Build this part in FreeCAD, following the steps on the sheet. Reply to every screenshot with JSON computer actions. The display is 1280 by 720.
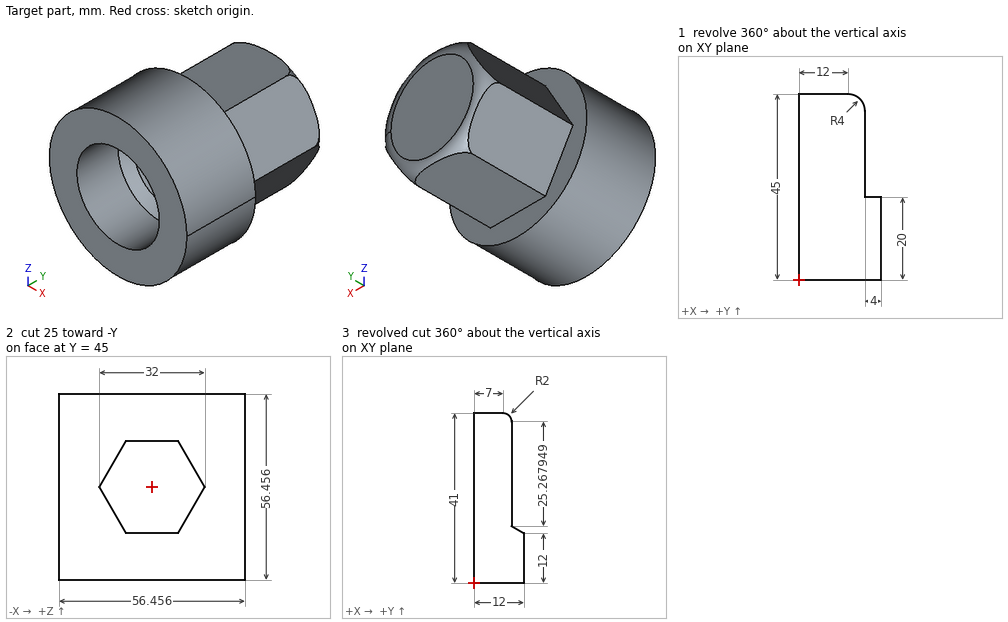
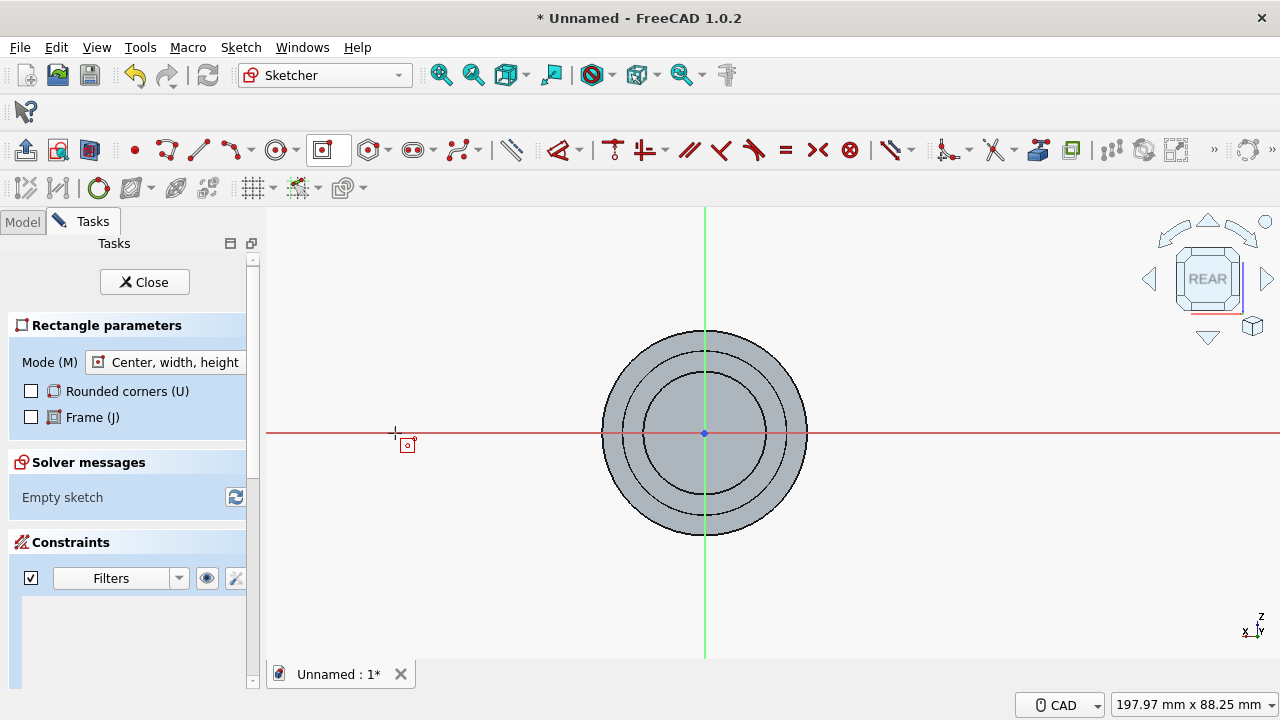
{"action": "left_click", "coordinate": [705, 433]}
{"action": "mouse_move", "coordinate": [849, 289]}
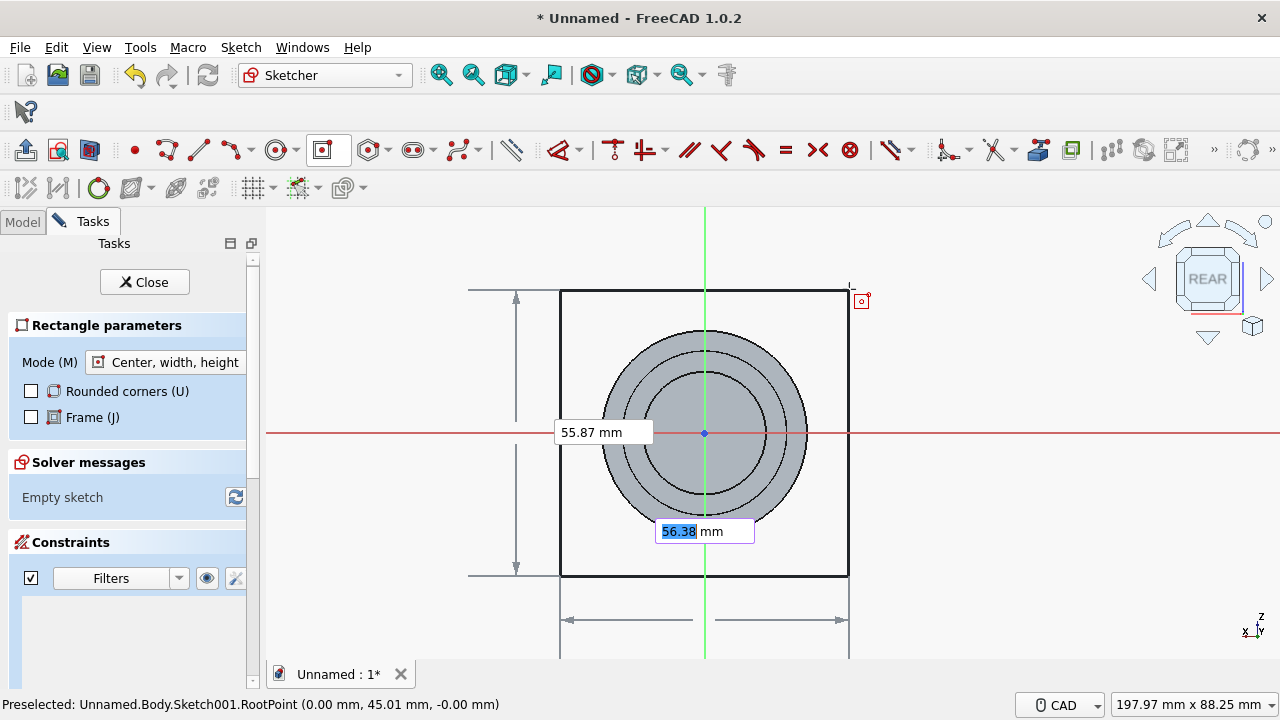
{"action": "type", "text": "56.456"}
{"action": "key", "text": "Tab"}
{"action": "type", "text": "56.456"}
{"action": "key", "text": "Return"}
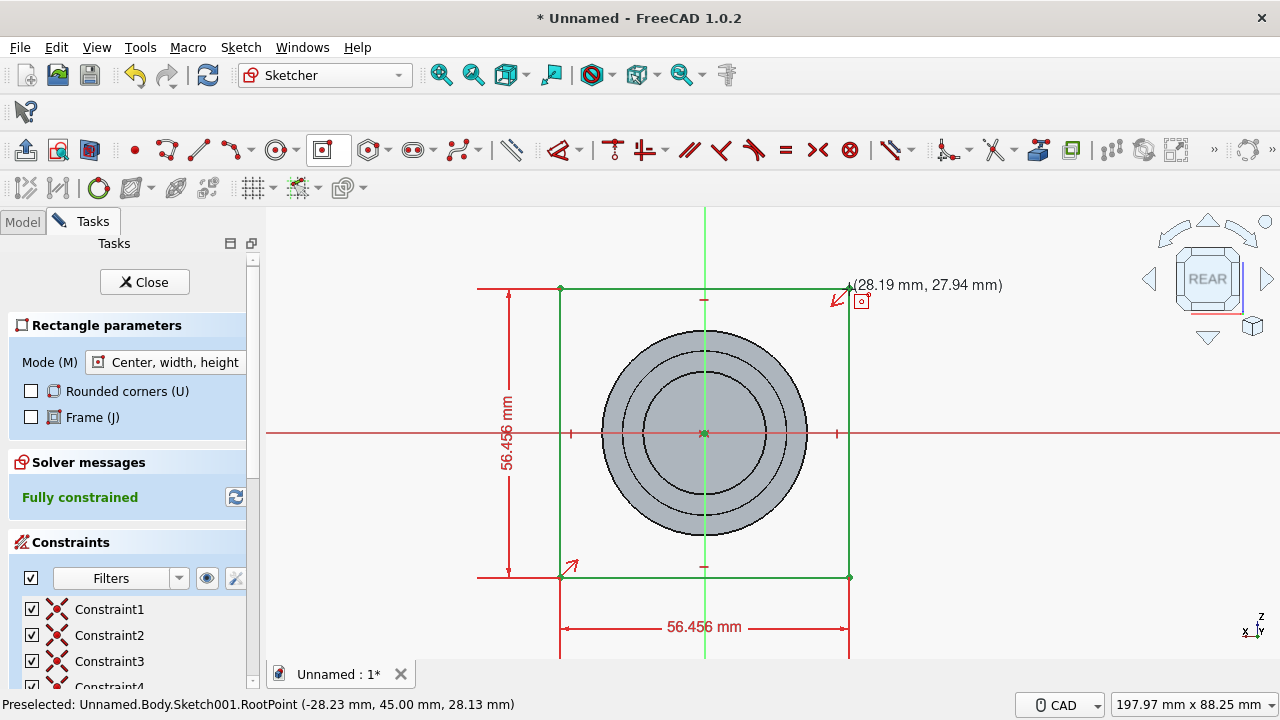
{"action": "key", "text": "g p 6"}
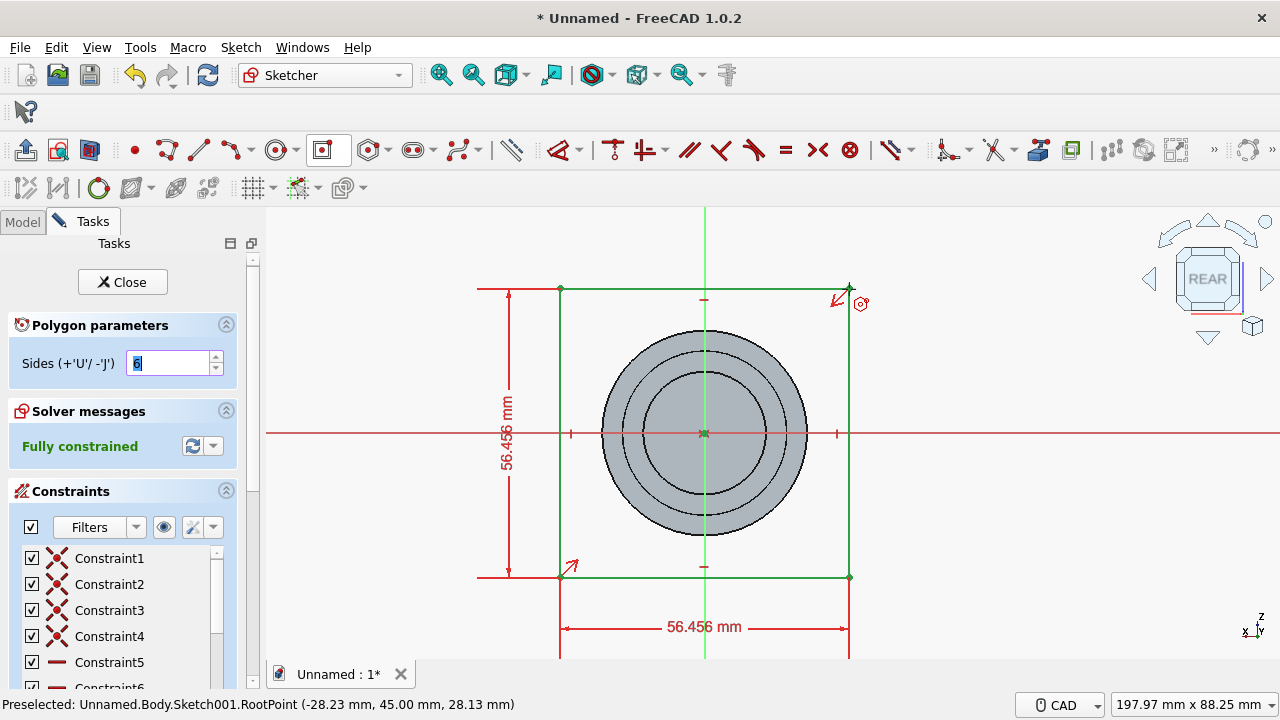
{"action": "left_click", "coordinate": [705, 433]}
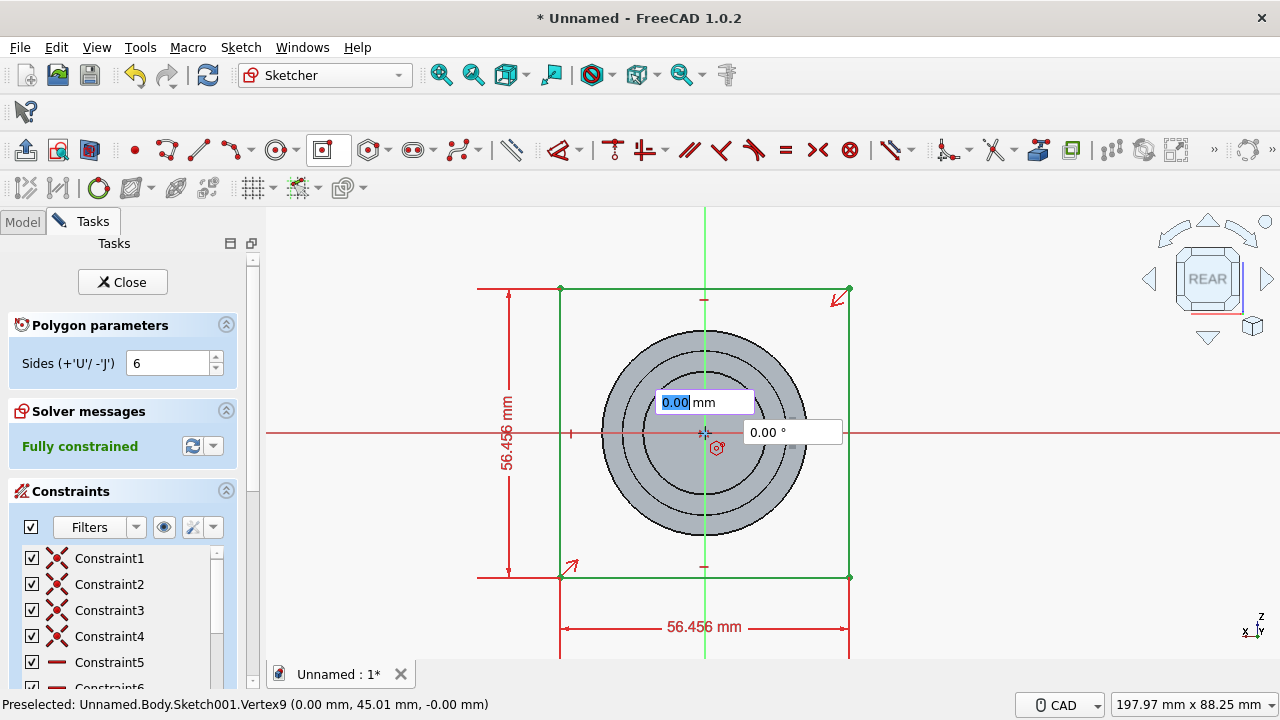
{"action": "left_click", "coordinate": [623, 433]}
{"action": "key", "text": "Escape"}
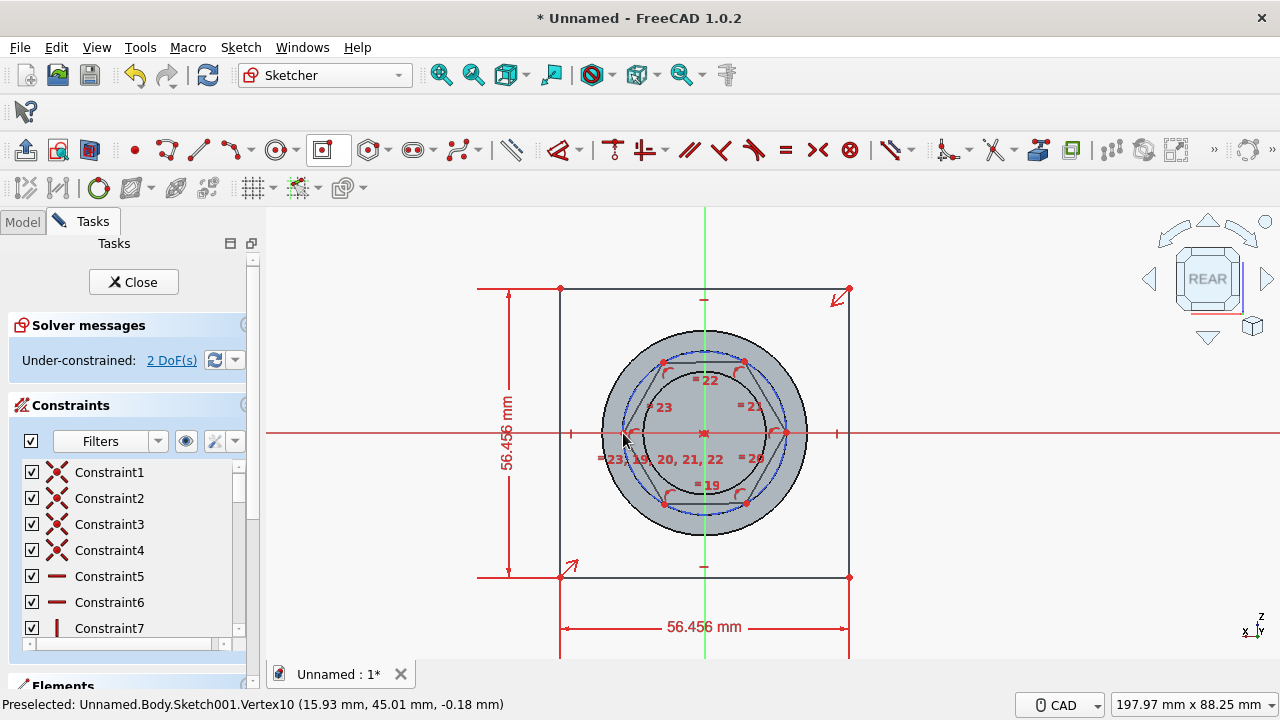
{"action": "scroll", "coordinate": [689, 504], "scroll_direction": "up", "scroll_amount": 3}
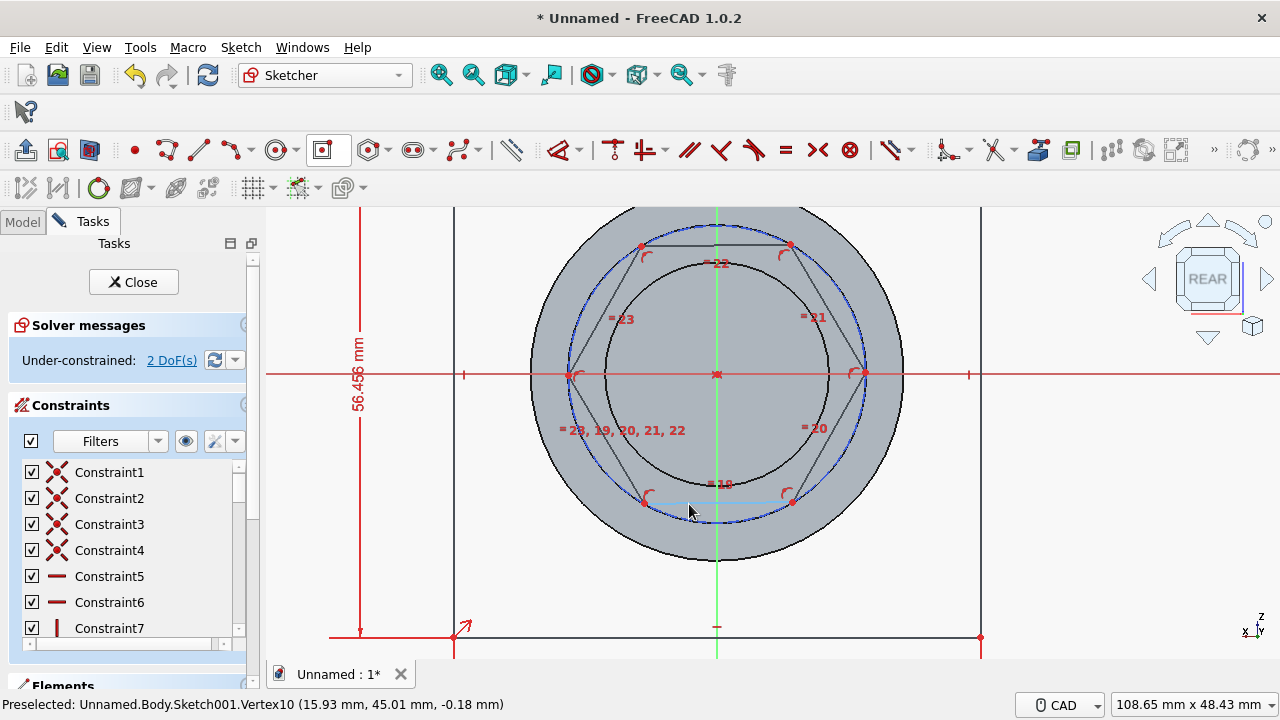
{"action": "left_click", "coordinate": [689, 503]}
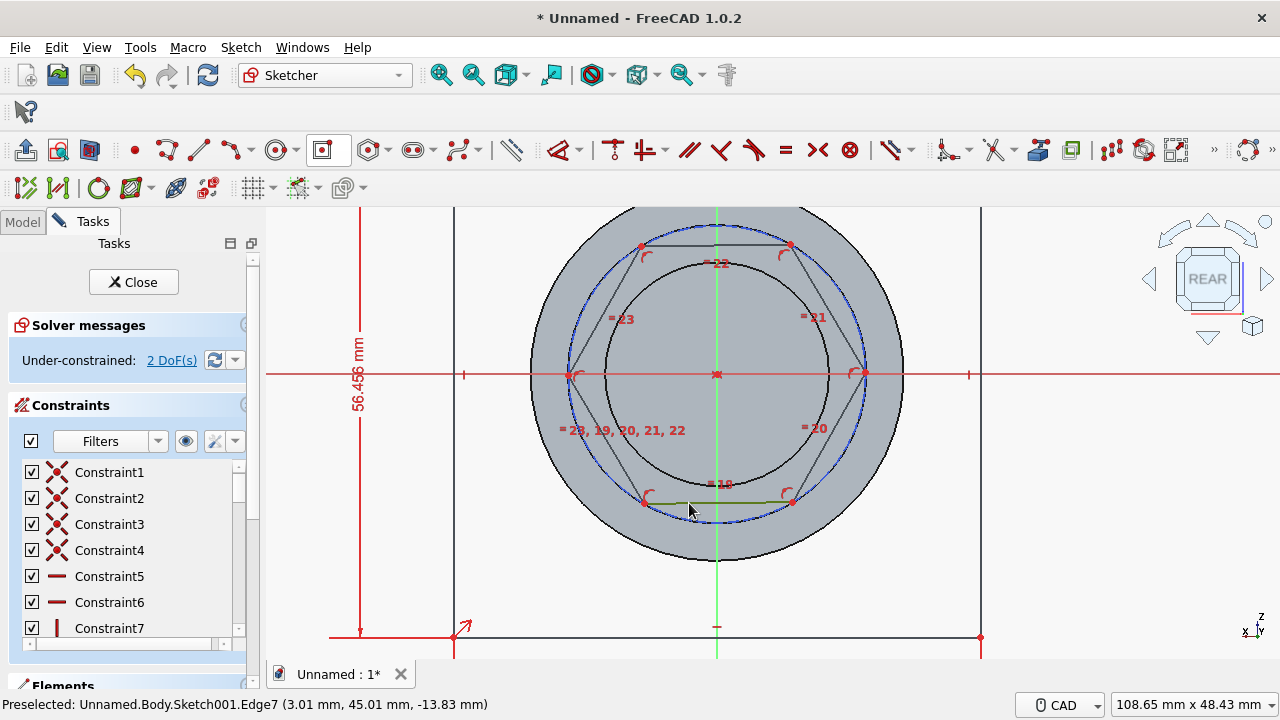
{"action": "left_click", "coordinate": [668, 150]}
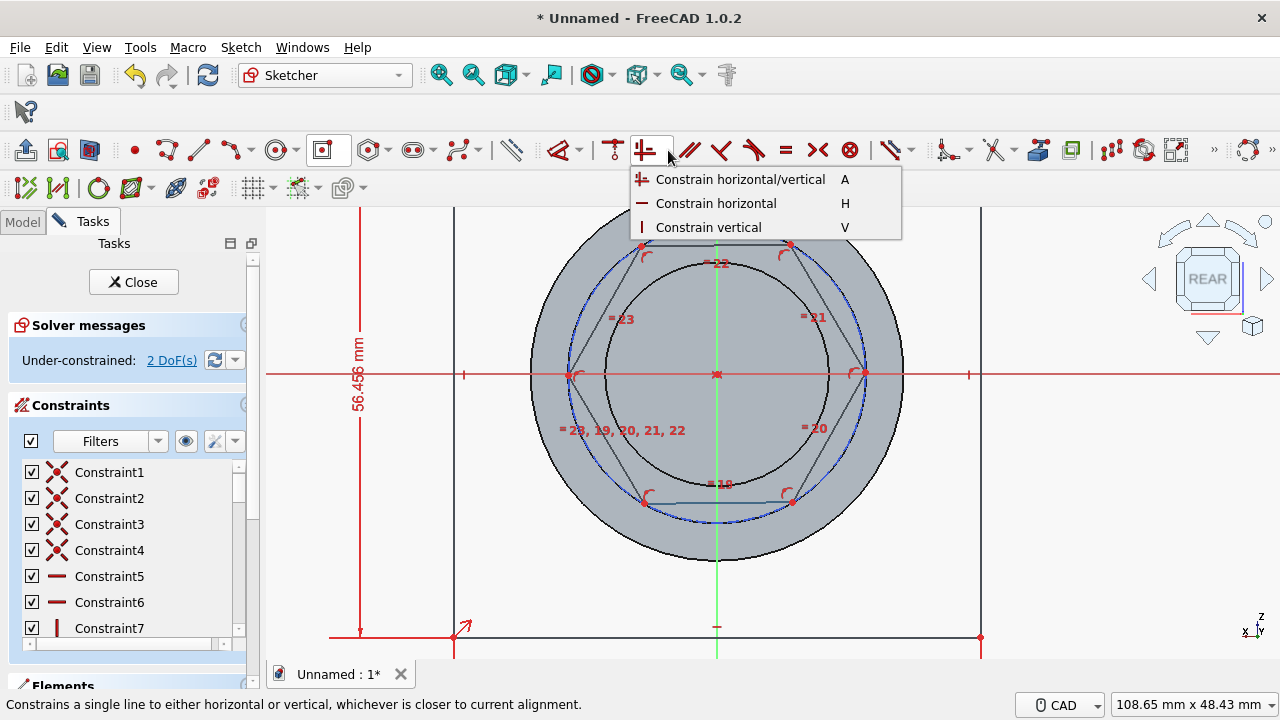
{"action": "left_click", "coordinate": [766, 203]}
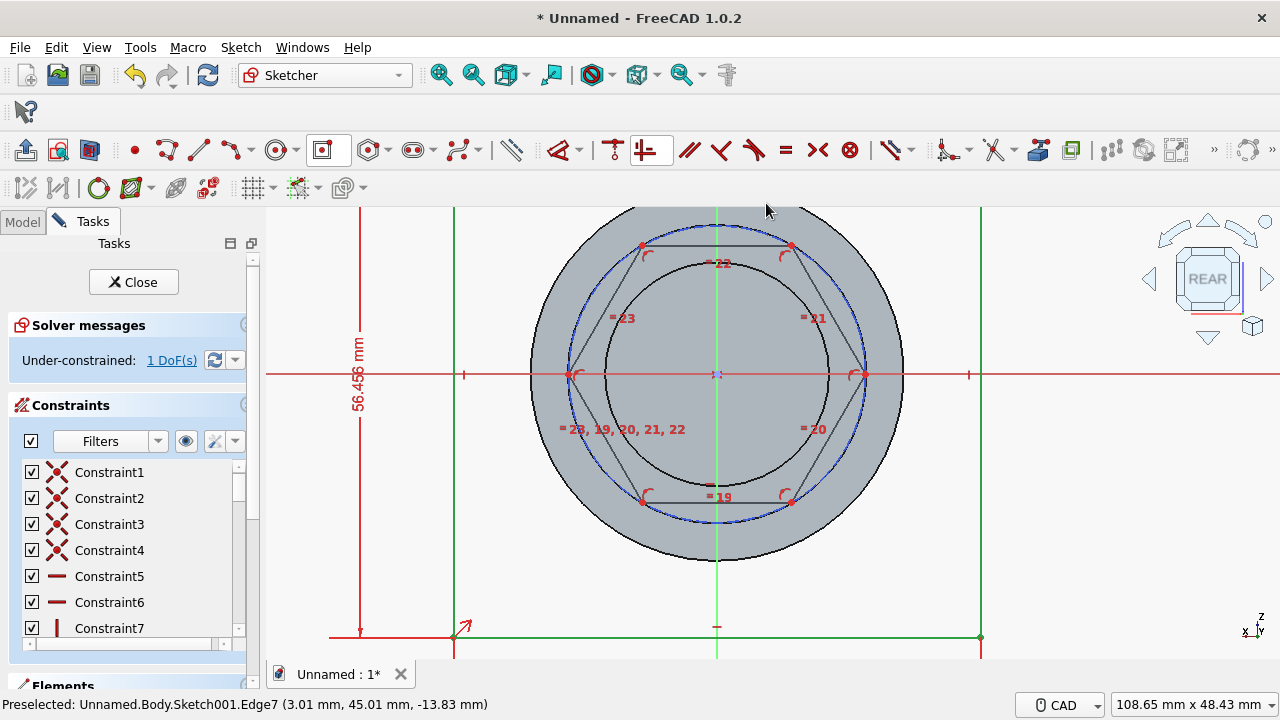
{"action": "key", "text": "d"}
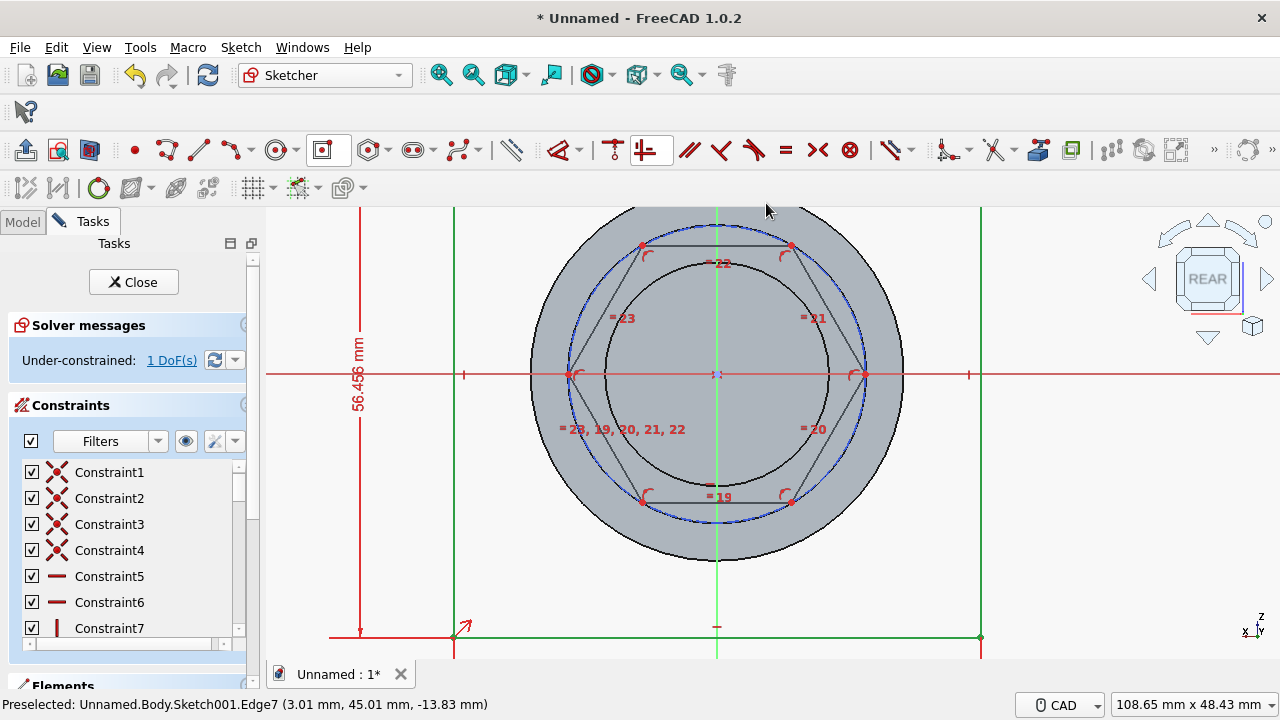
{"action": "left_click", "coordinate": [568, 374]}